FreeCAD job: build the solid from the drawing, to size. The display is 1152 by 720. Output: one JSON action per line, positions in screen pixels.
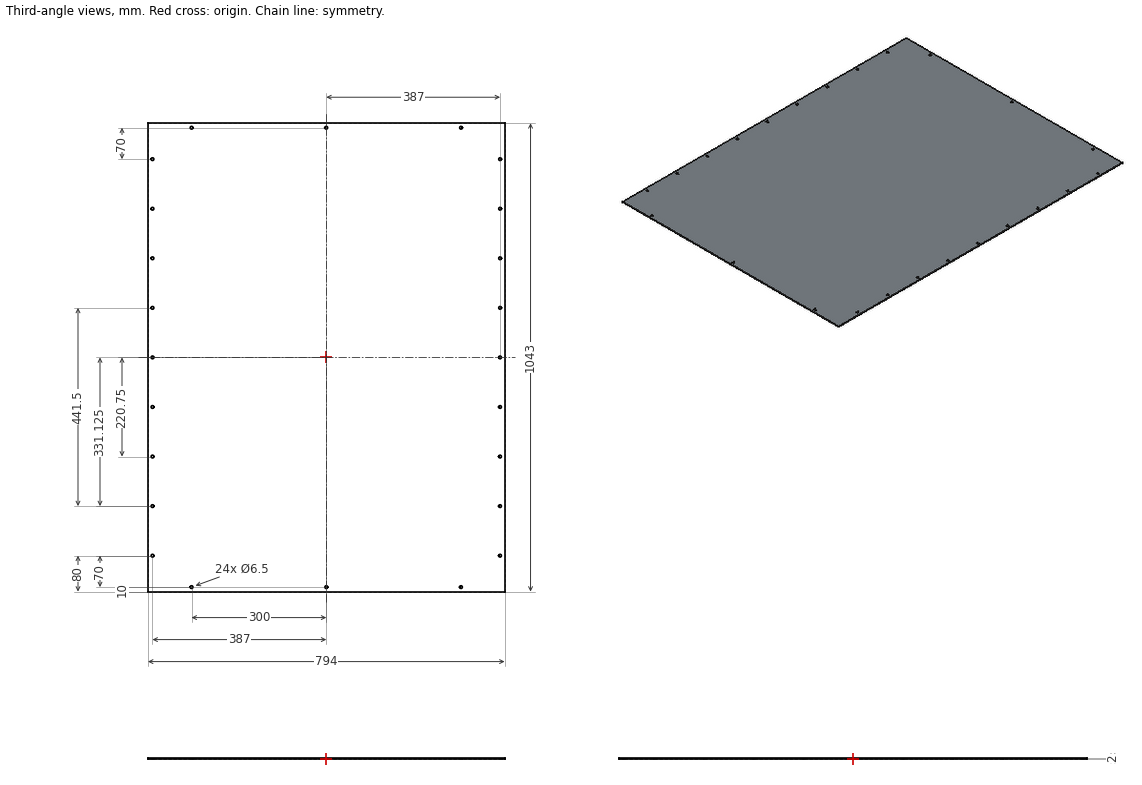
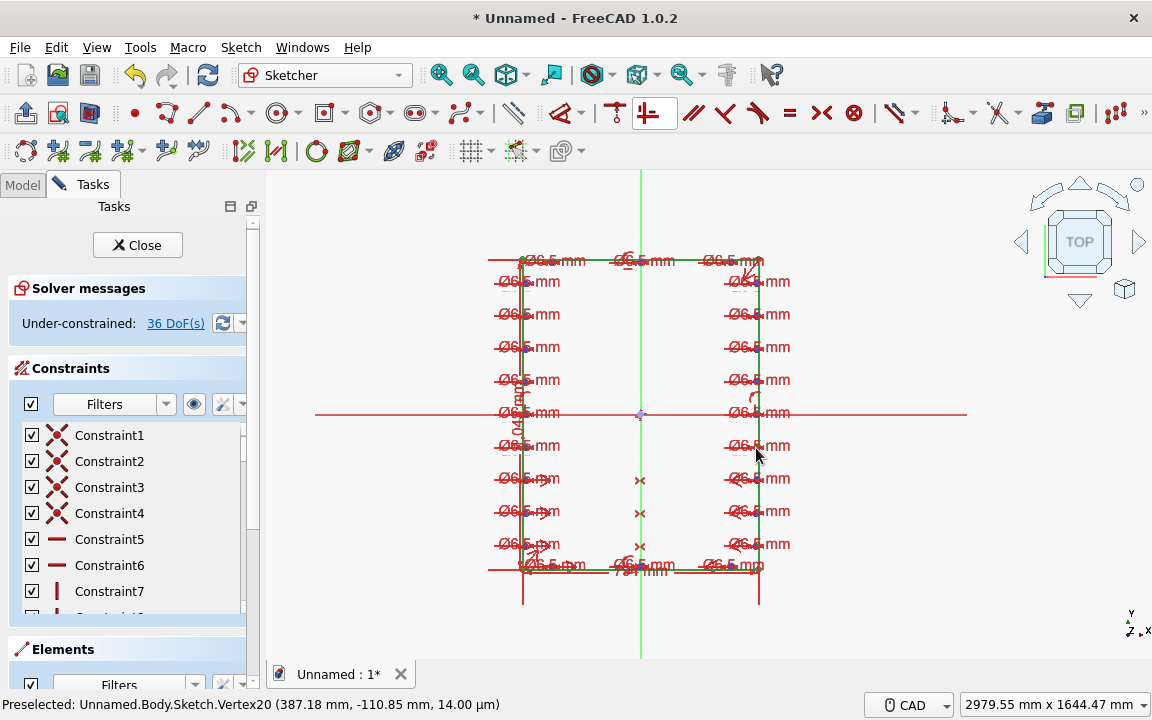
{"action": "left_click", "coordinate": [641, 600]}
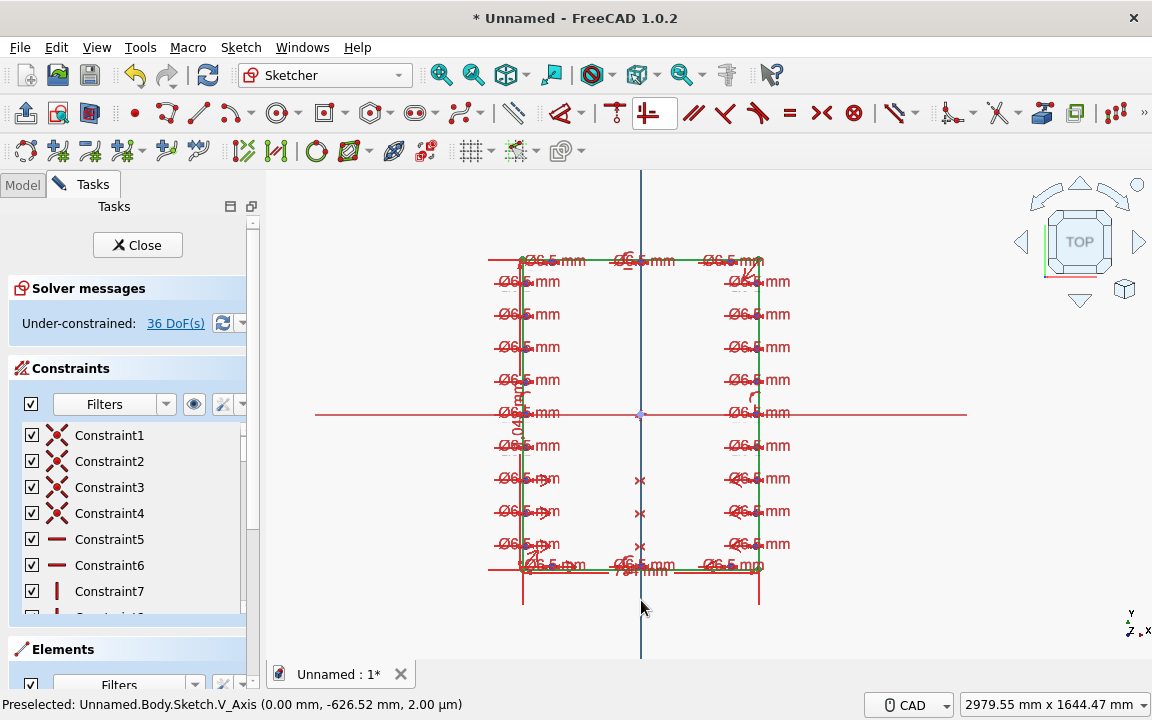
{"action": "left_click", "coordinate": [822, 114]}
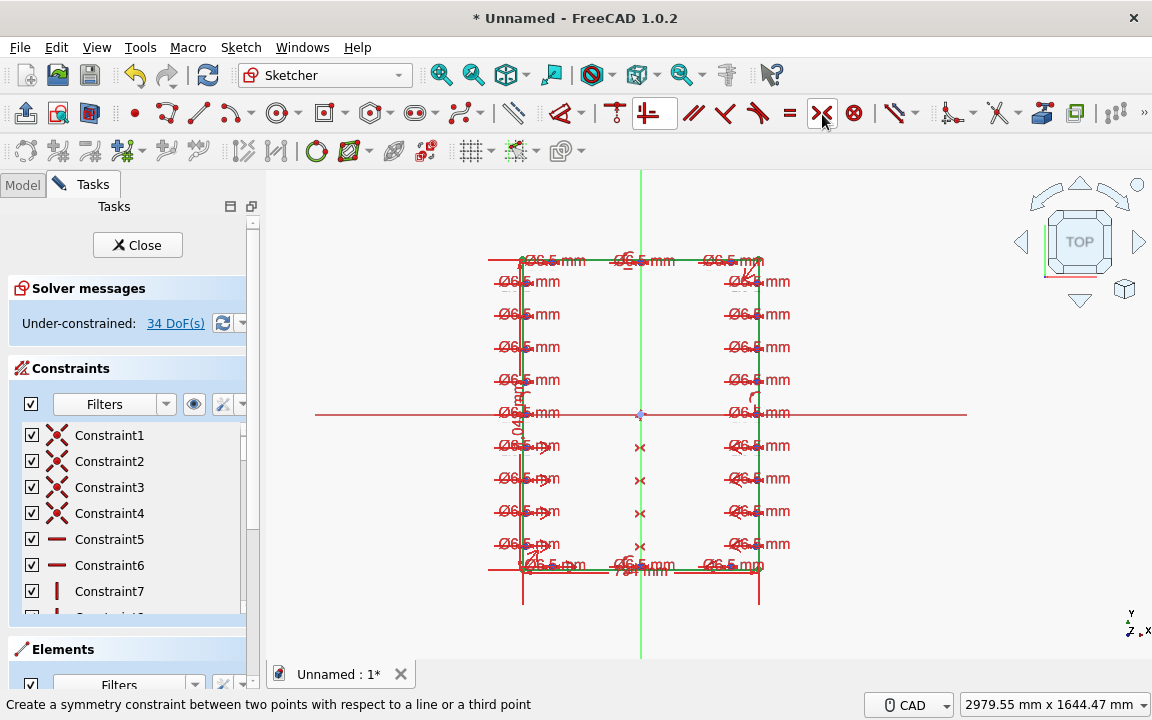
{"action": "left_click", "coordinate": [526, 448]}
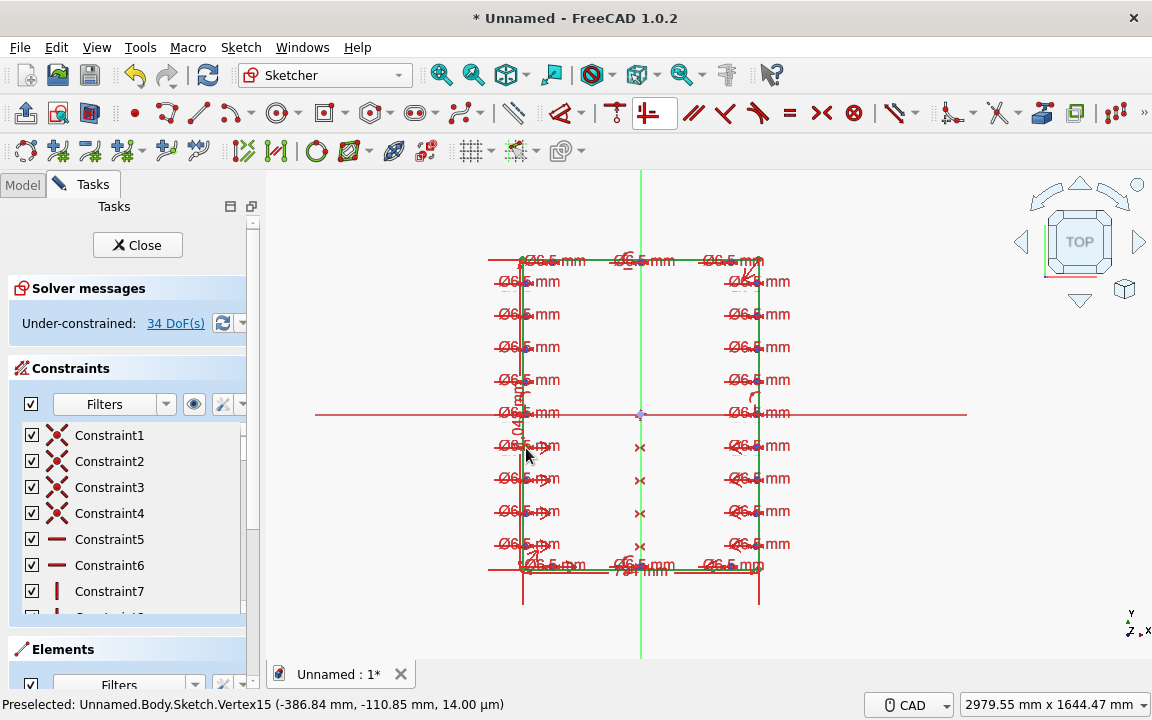
{"action": "left_click", "coordinate": [526, 382]}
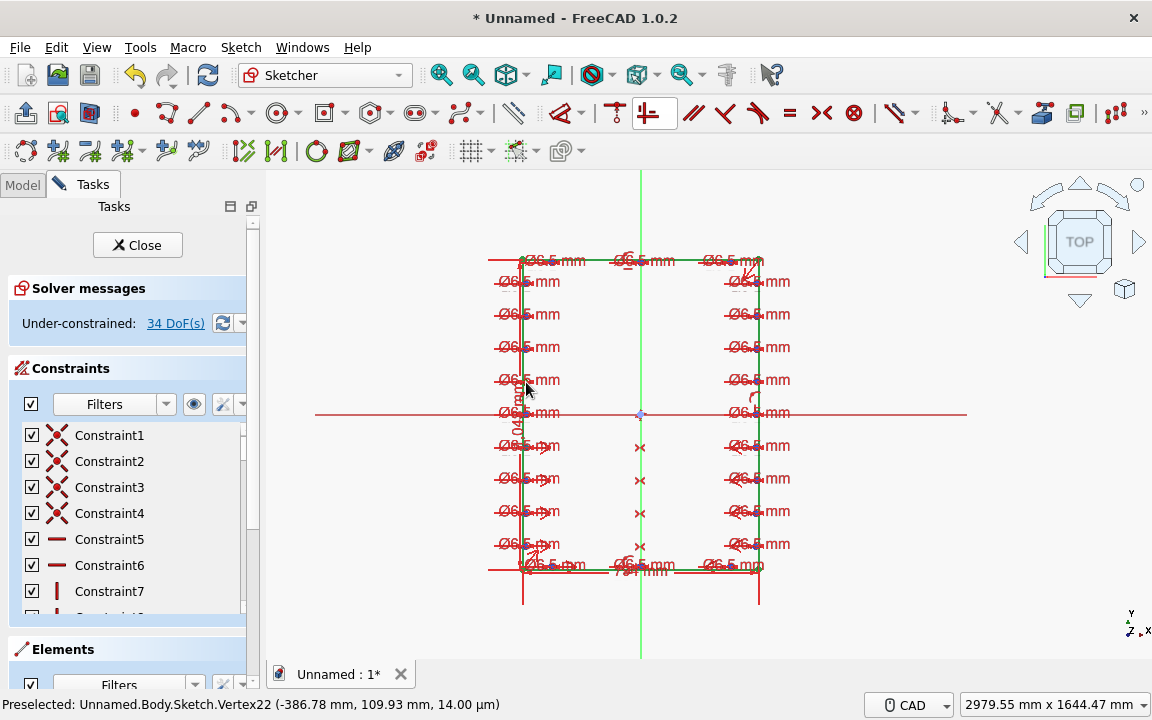
{"action": "left_click", "coordinate": [344, 415]}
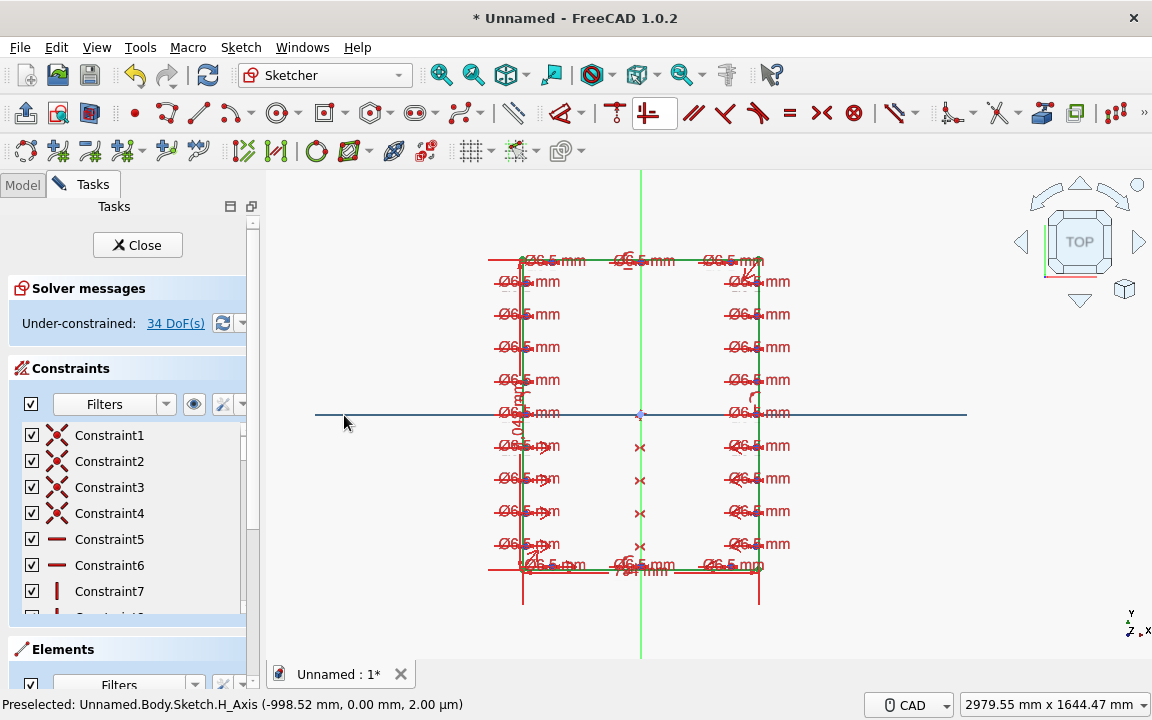
{"action": "left_click", "coordinate": [822, 114]}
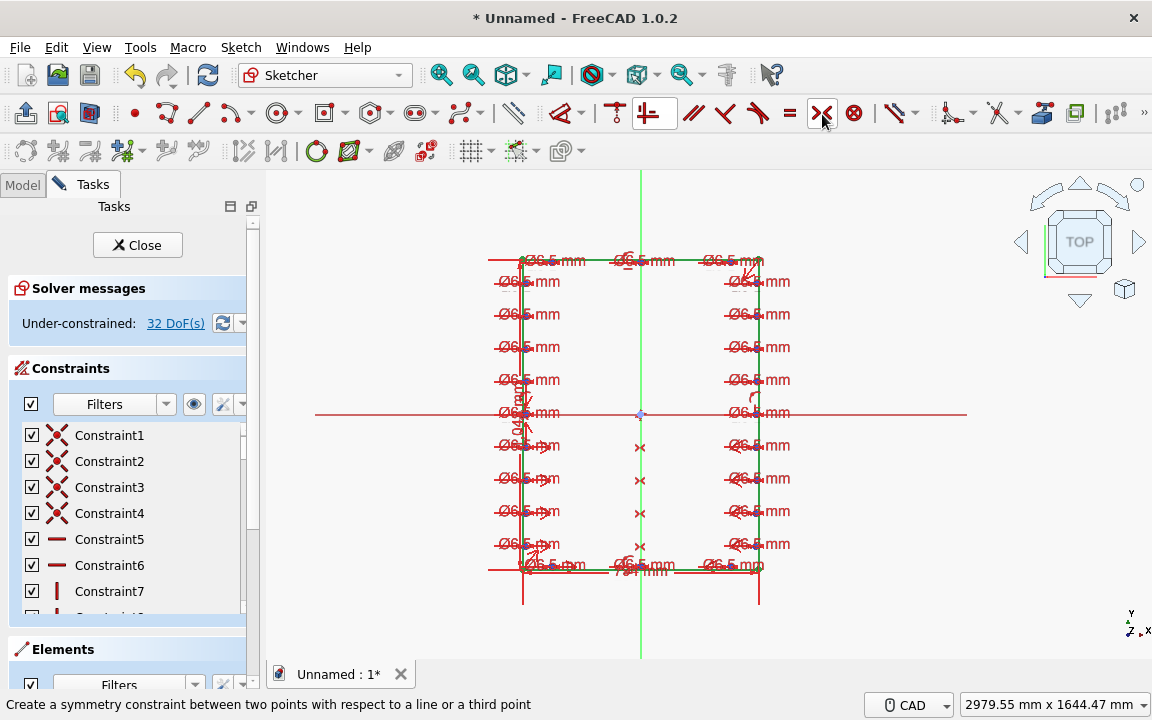
{"action": "left_click", "coordinate": [526, 480]}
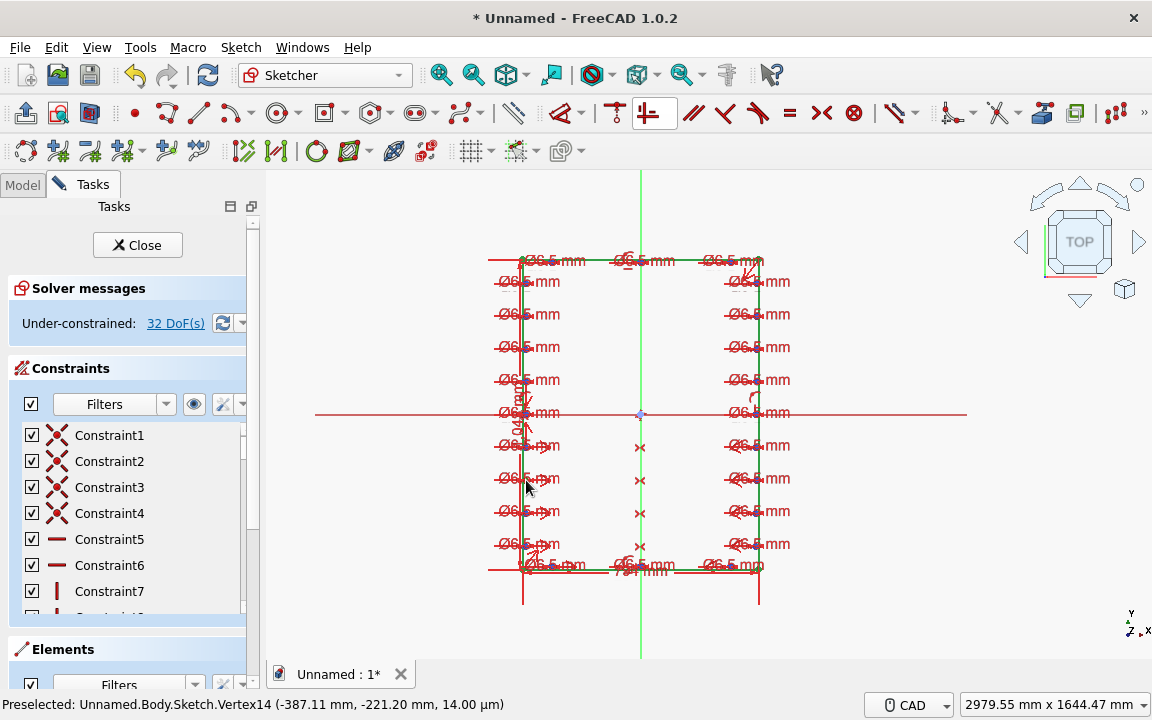
{"action": "left_click", "coordinate": [526, 349]}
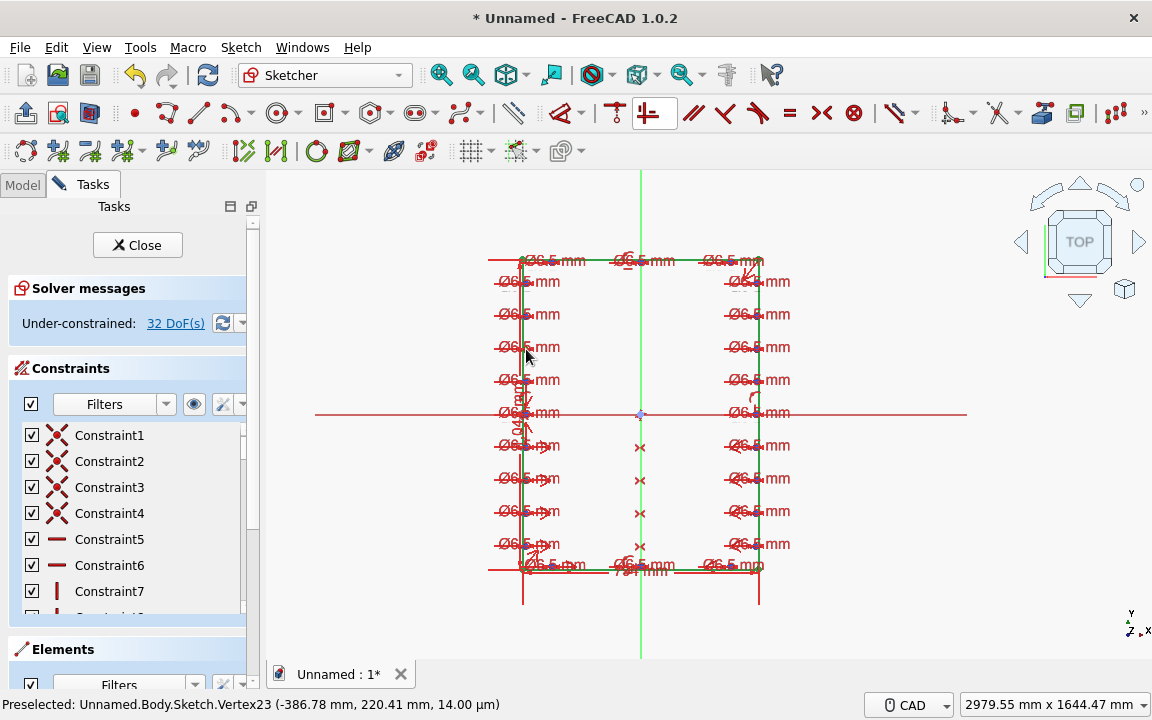
{"action": "left_click", "coordinate": [344, 415]}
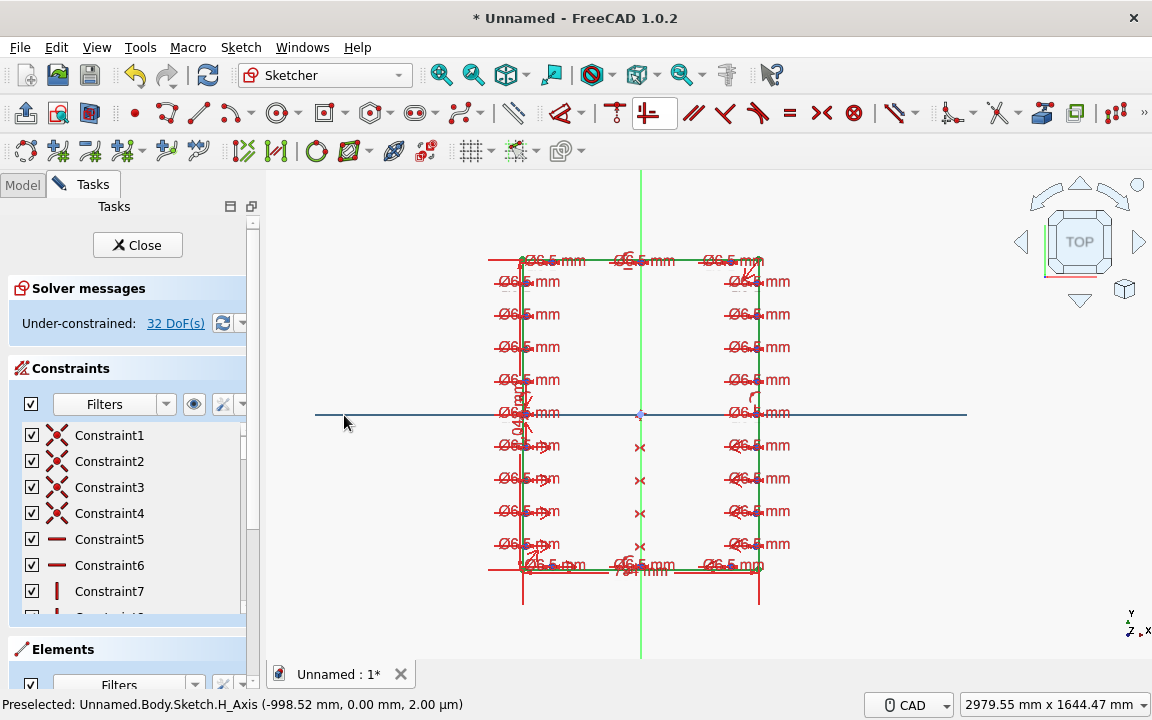
{"action": "left_click", "coordinate": [822, 114]}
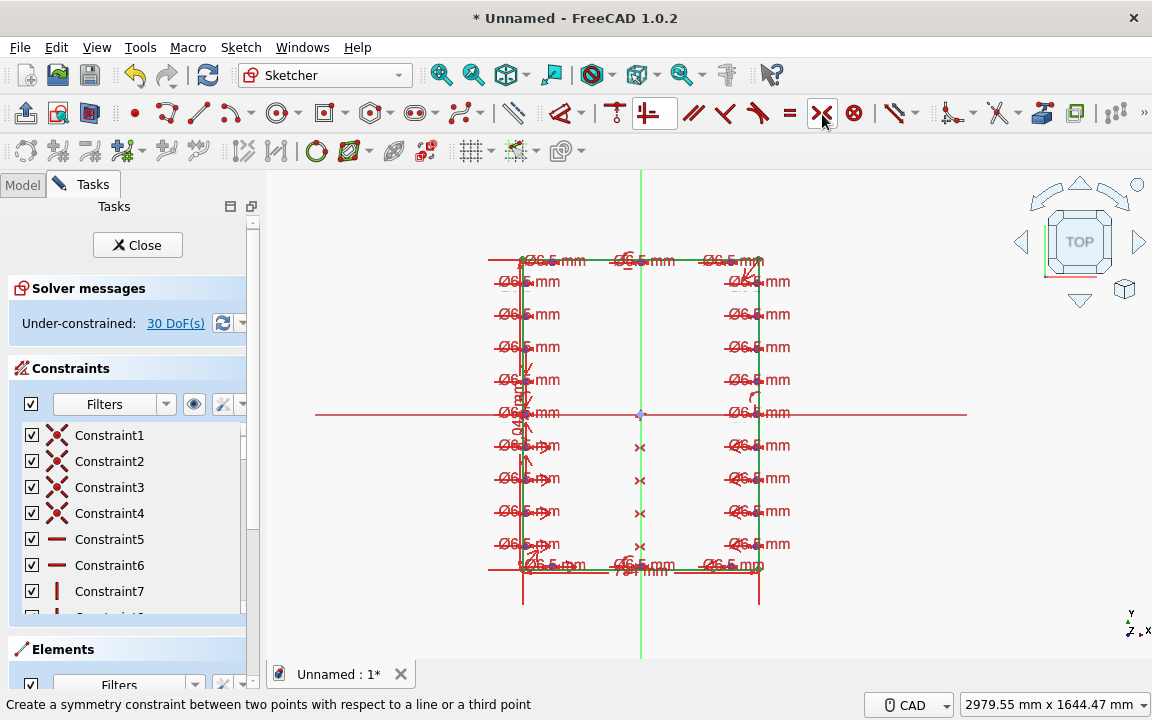
{"action": "left_click", "coordinate": [526, 513]}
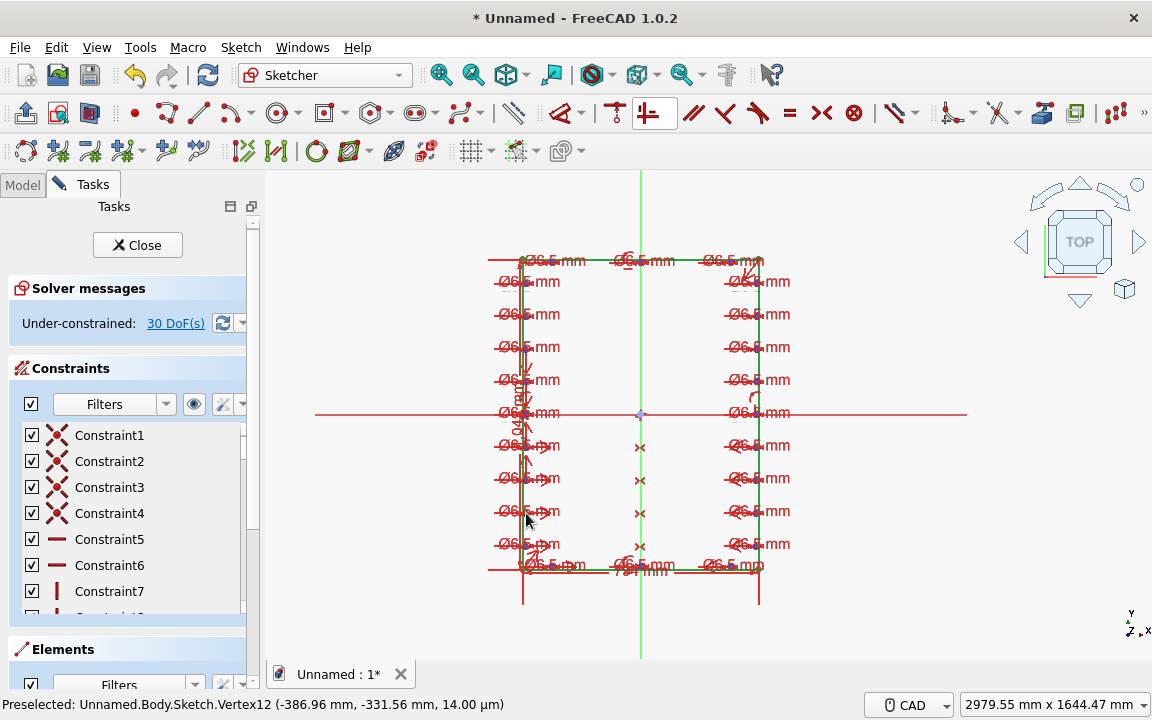
{"action": "left_click", "coordinate": [526, 316]}